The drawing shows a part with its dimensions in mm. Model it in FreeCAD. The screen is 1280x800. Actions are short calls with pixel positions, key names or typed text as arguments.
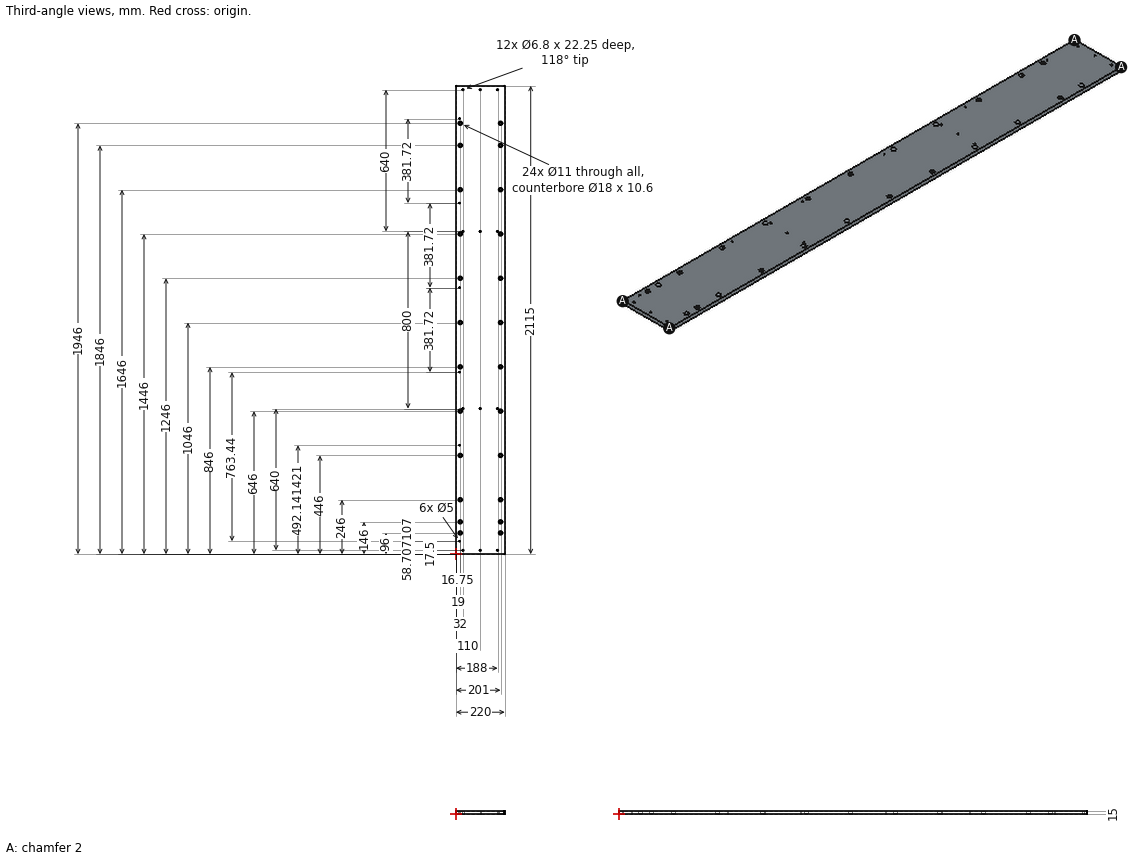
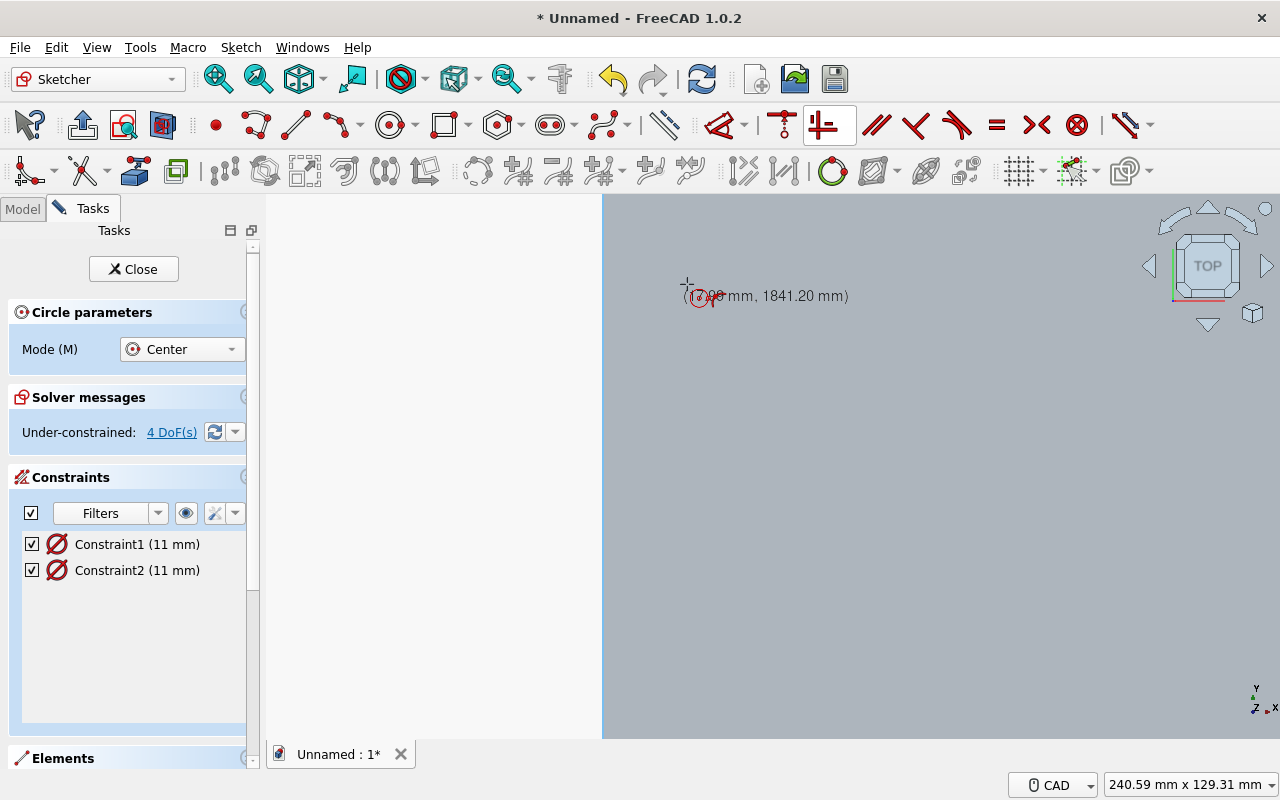
scroll(687, 284, down, 15)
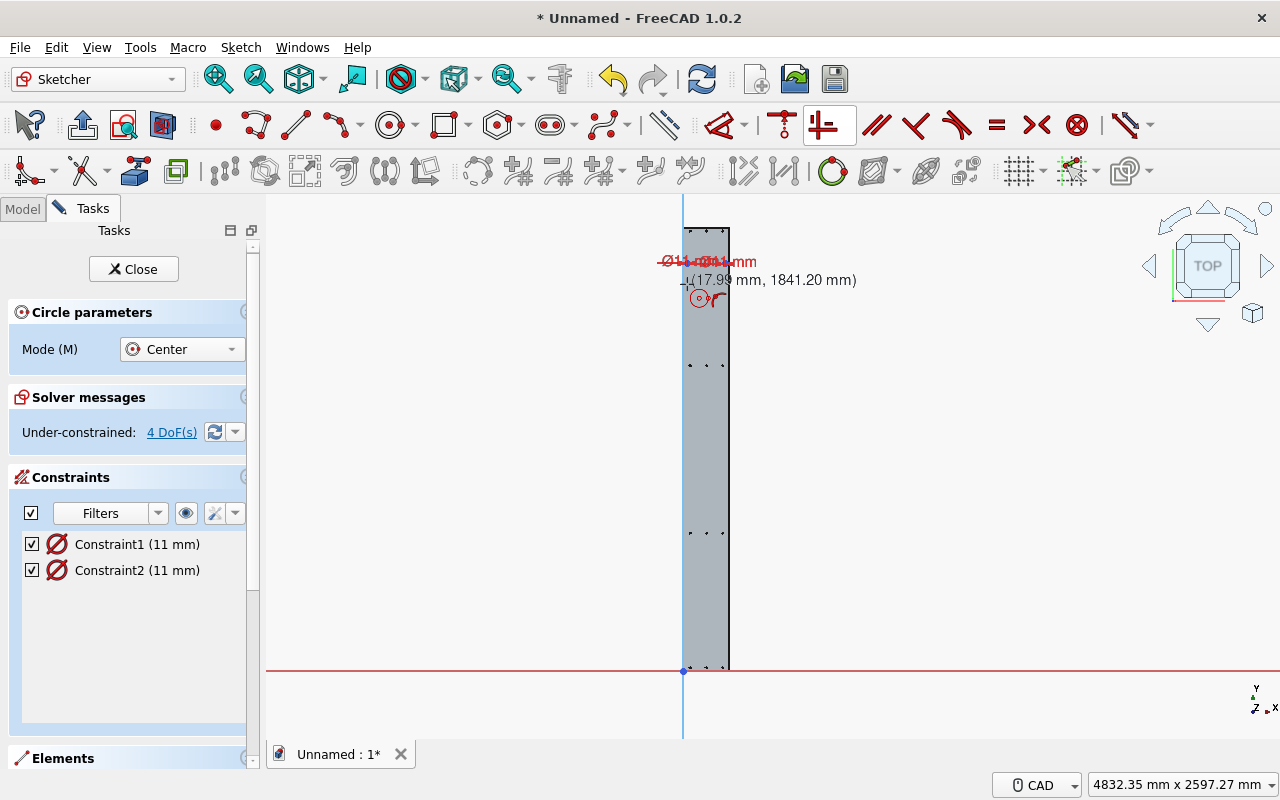
scroll(687, 284, up, 7)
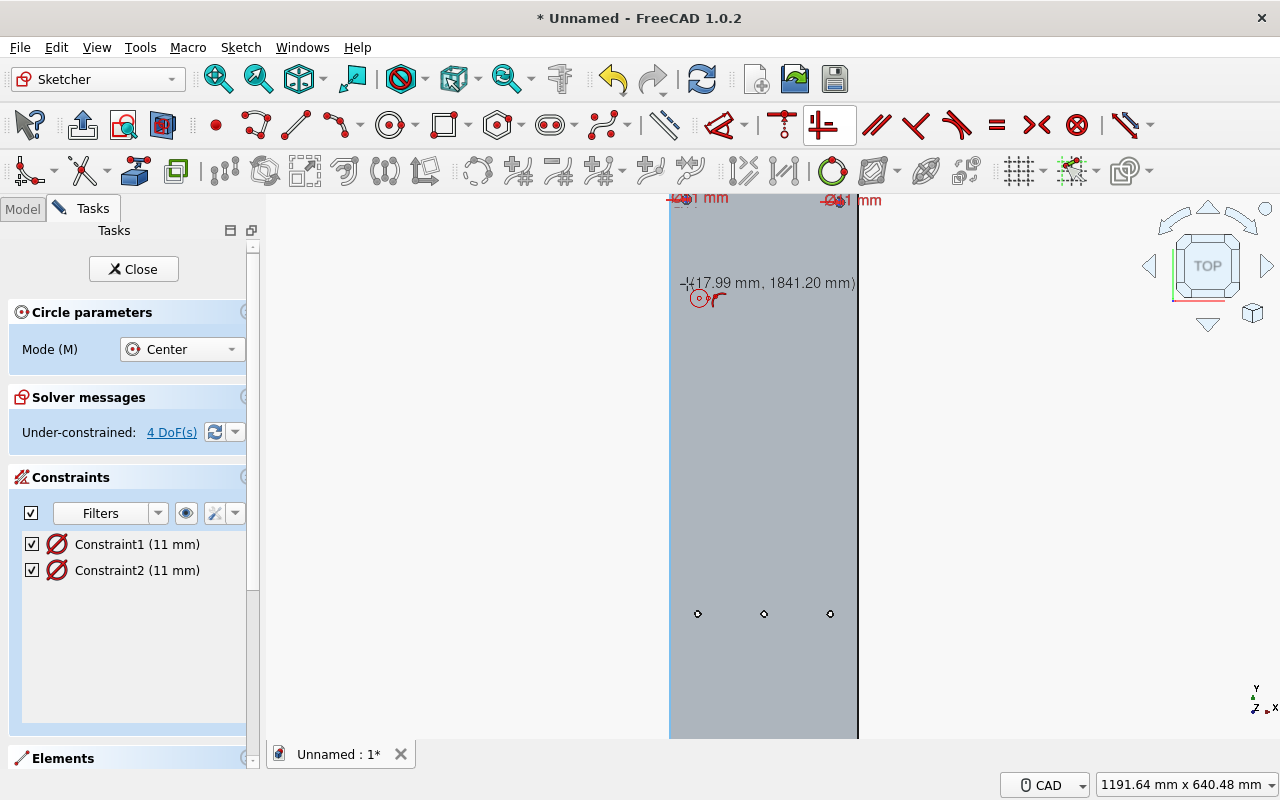
click(687, 283)
move(690, 280)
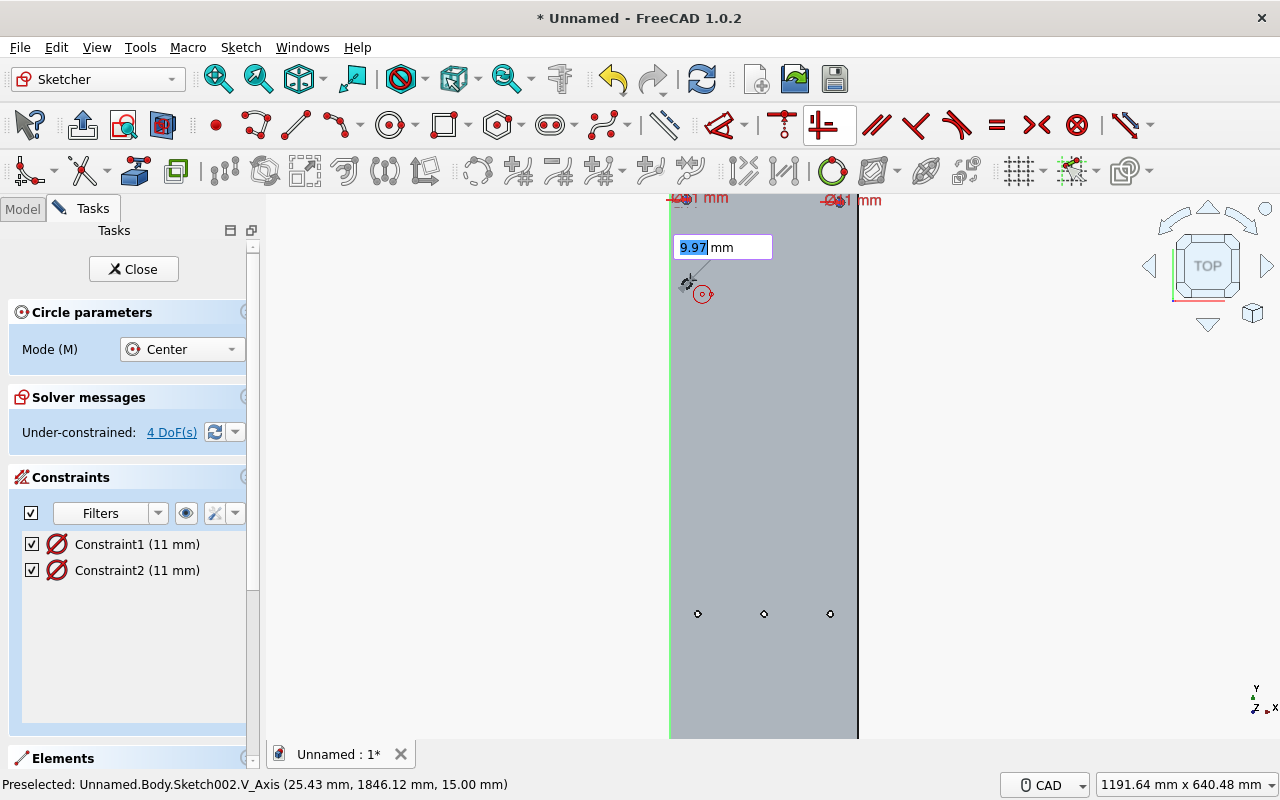
text(11)
key(Return)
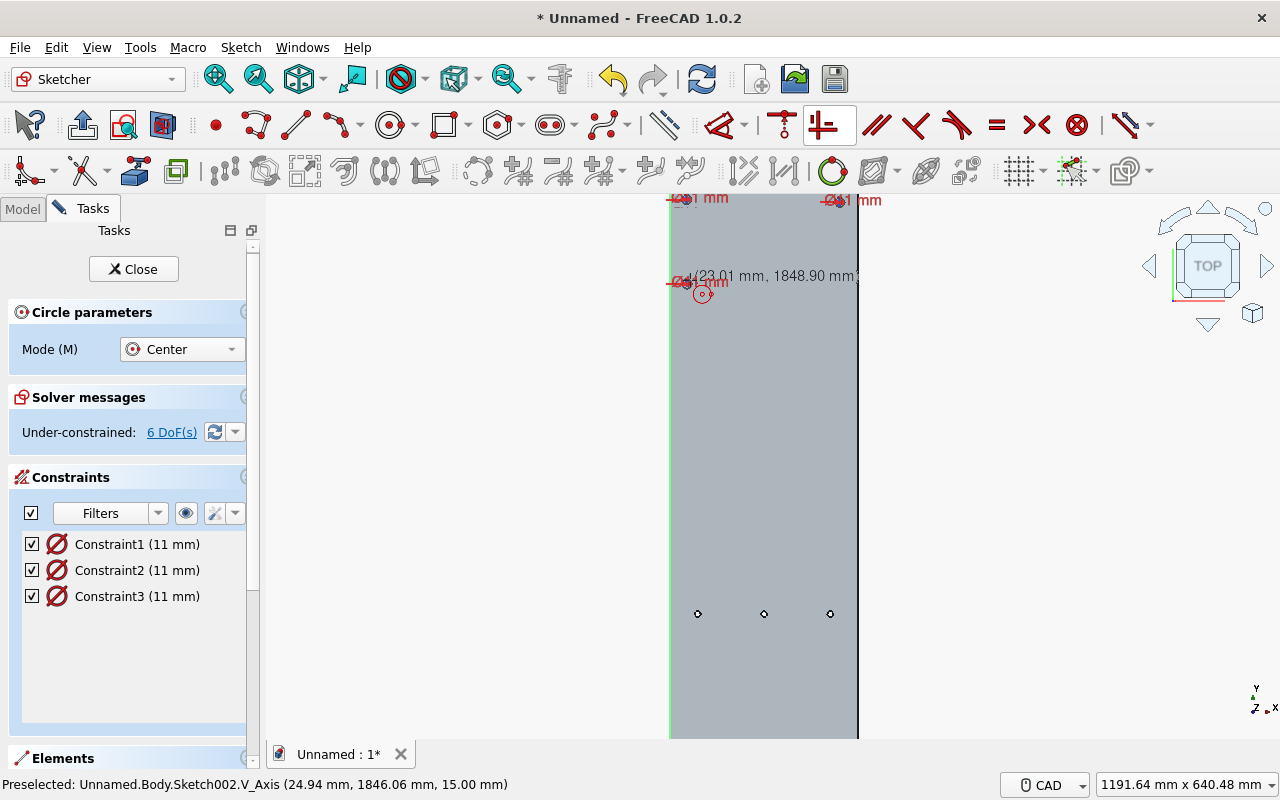
scroll(841, 283, up, 8)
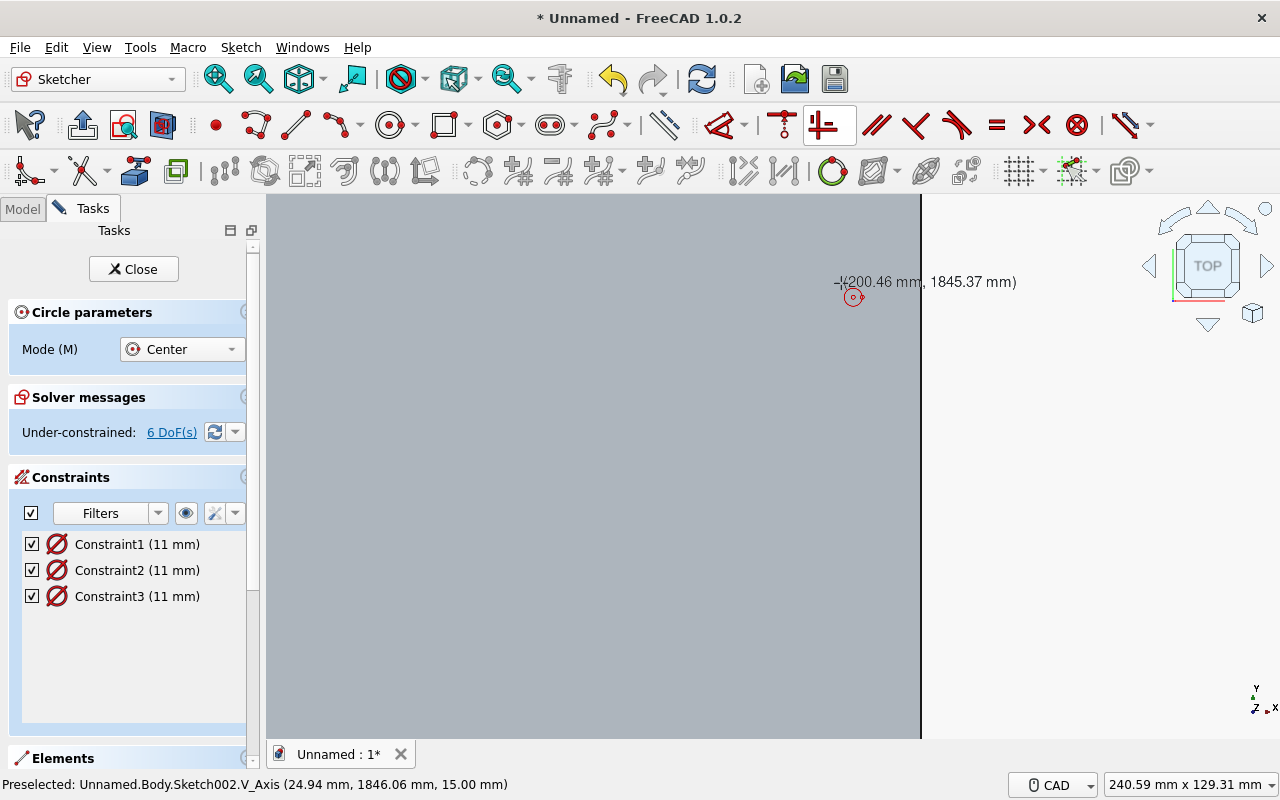
scroll(719, 284, down, 15)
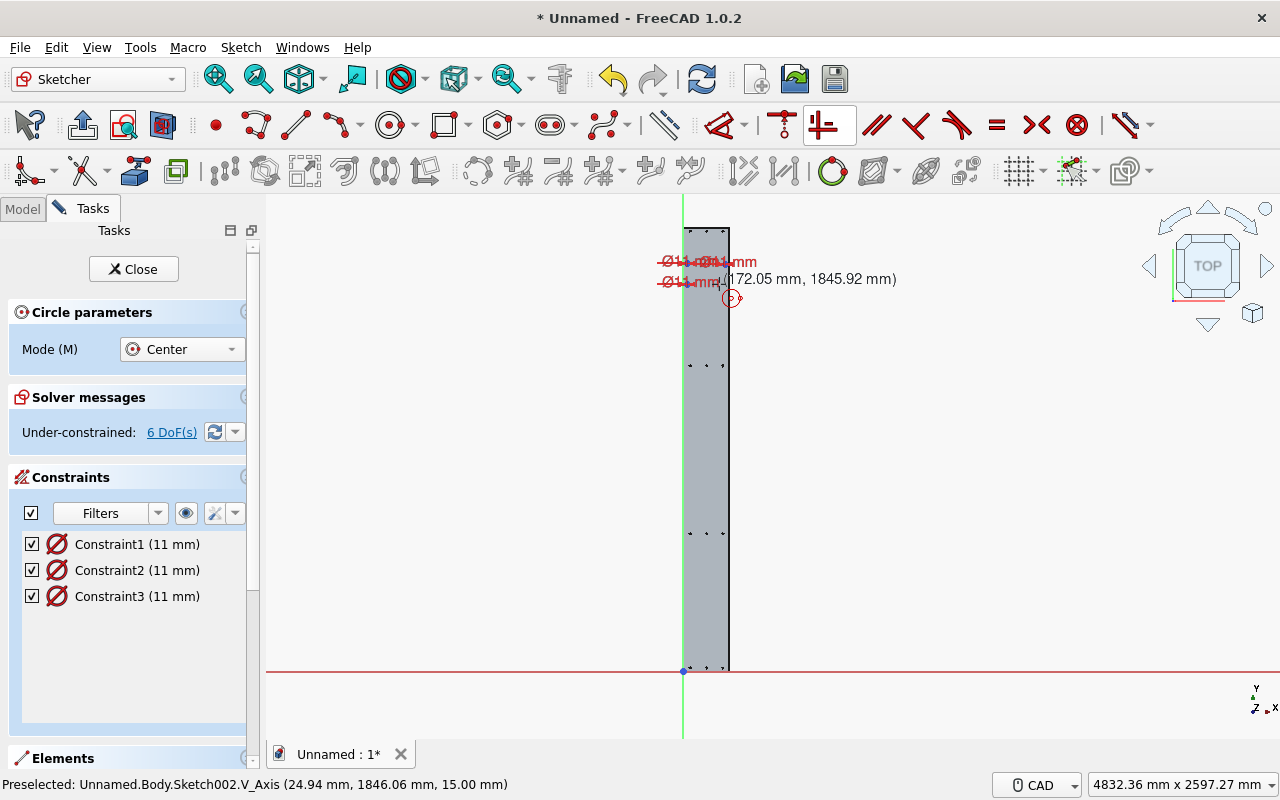
click(726, 284)
move(726, 283)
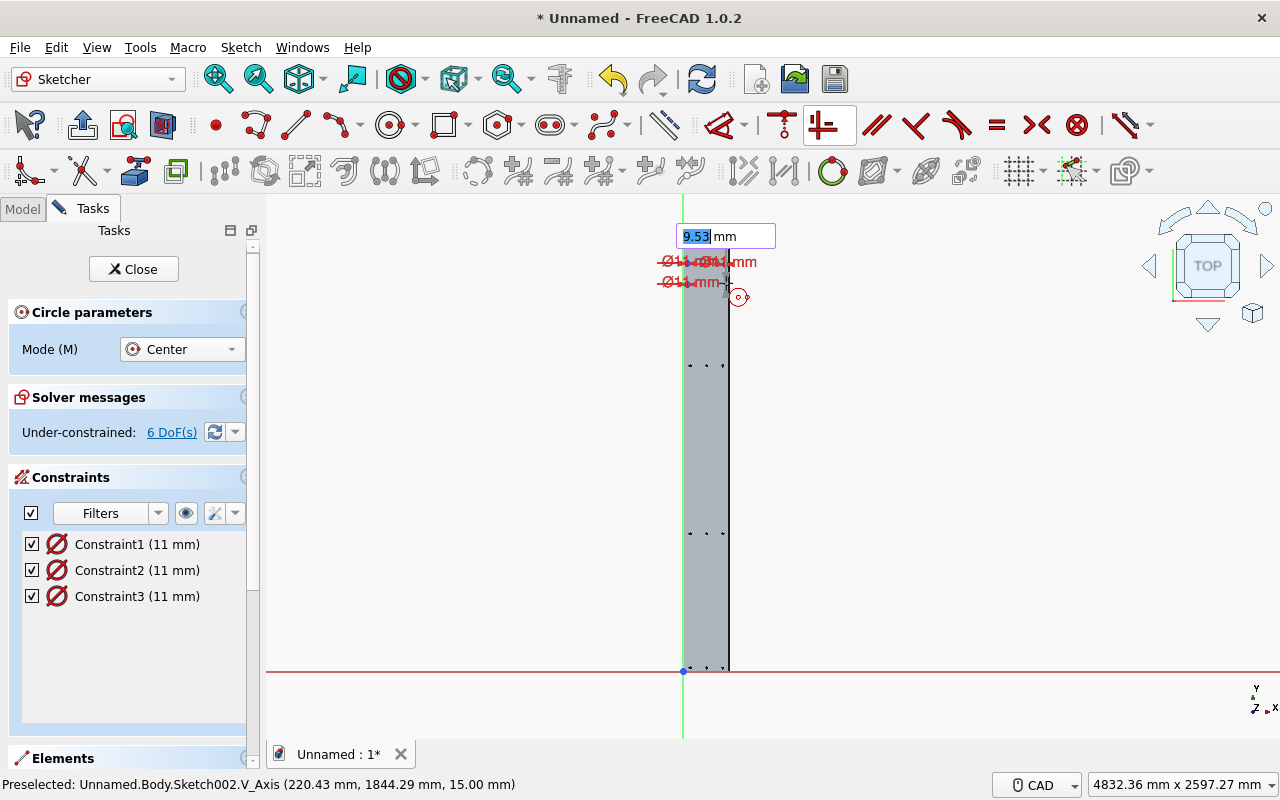
text(11)
key(Return)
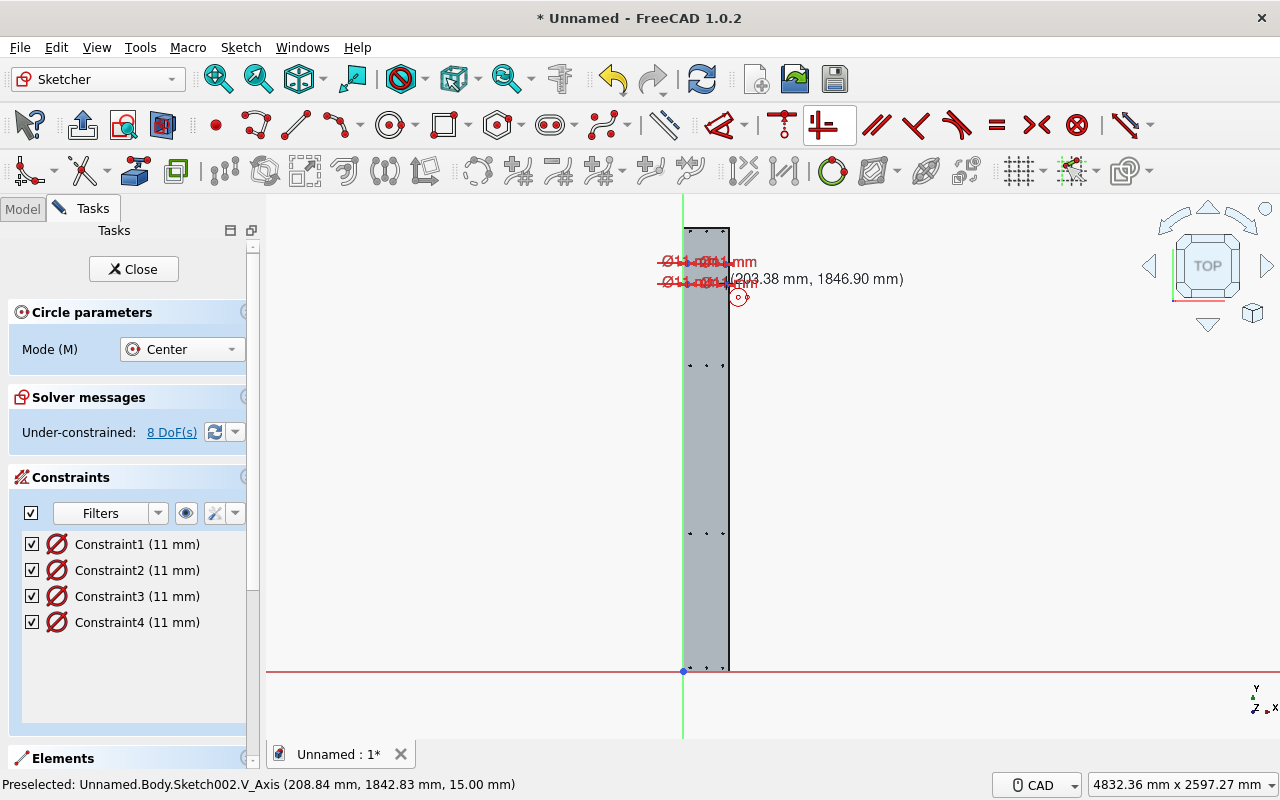
scroll(687, 326, up, 15)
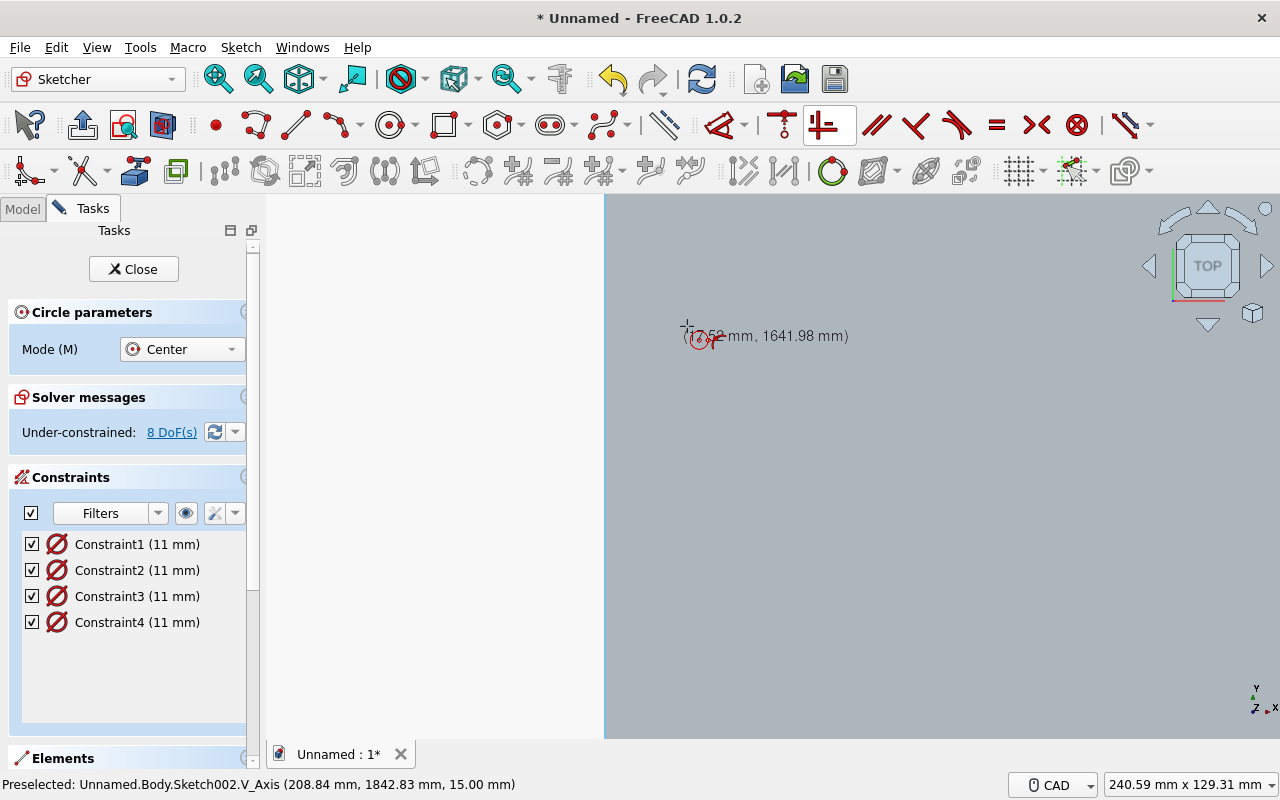
scroll(687, 326, down, 15)